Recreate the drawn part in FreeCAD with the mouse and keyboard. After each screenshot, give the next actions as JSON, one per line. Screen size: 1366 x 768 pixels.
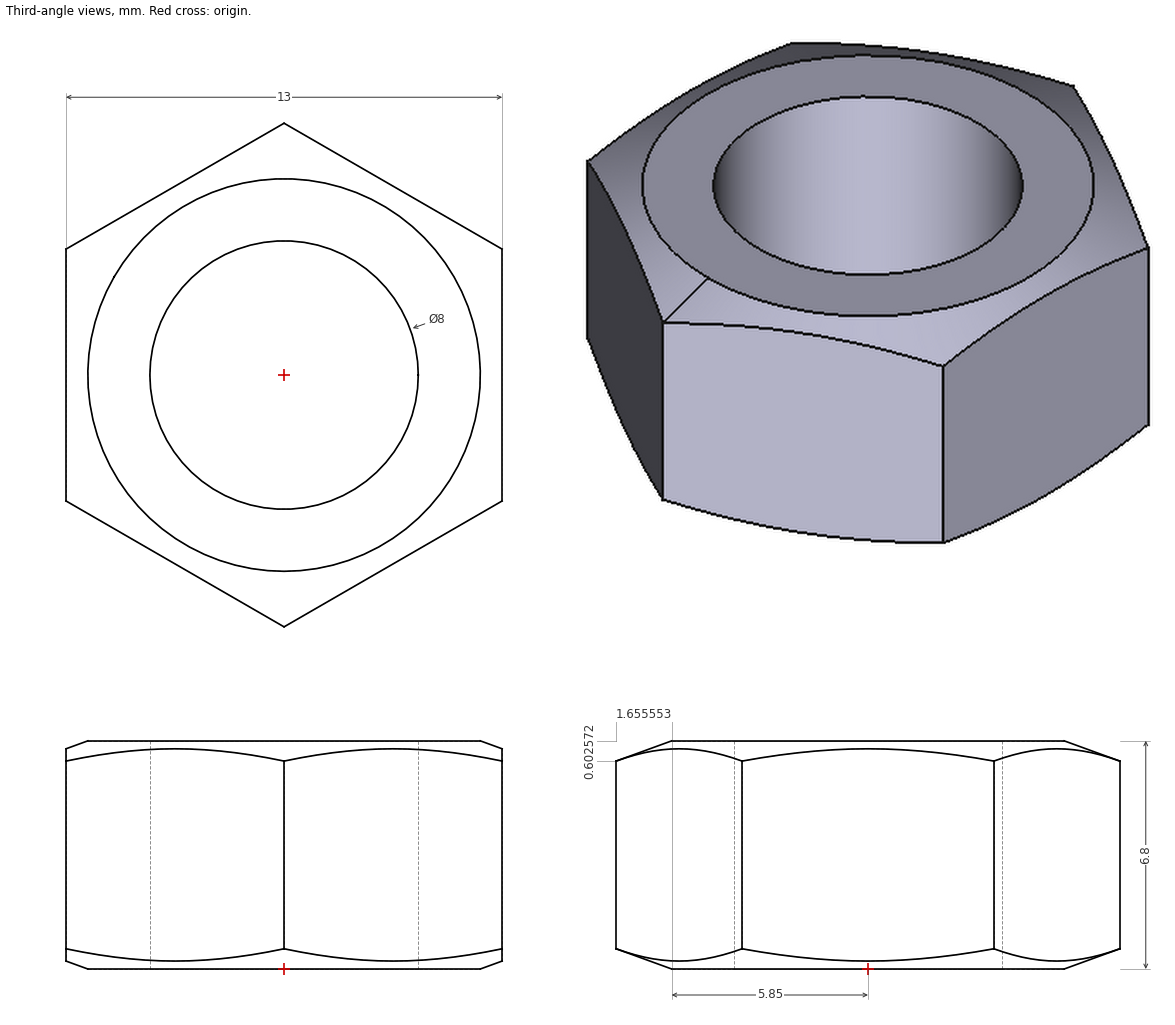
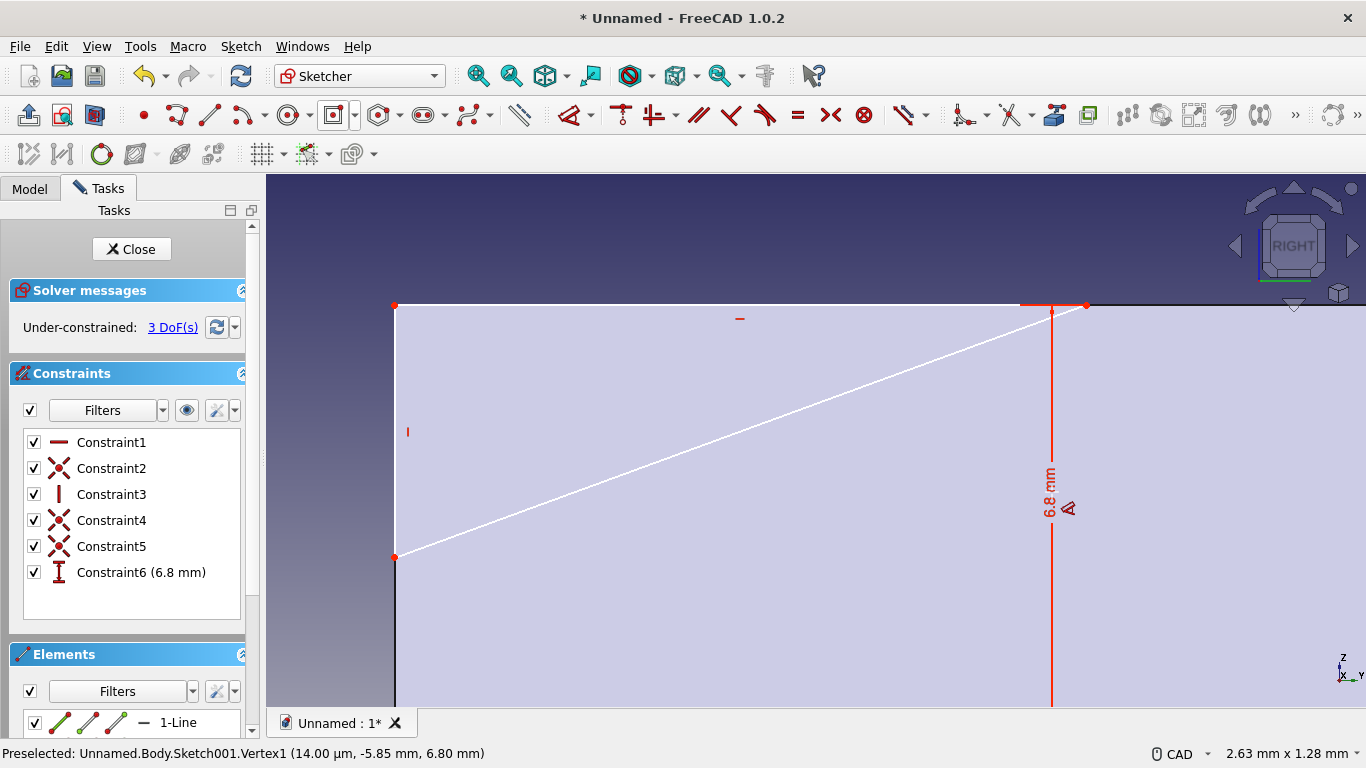
{"action": "left_click", "coordinate": [1086, 305]}
{"action": "left_click", "coordinate": [1143, 271]}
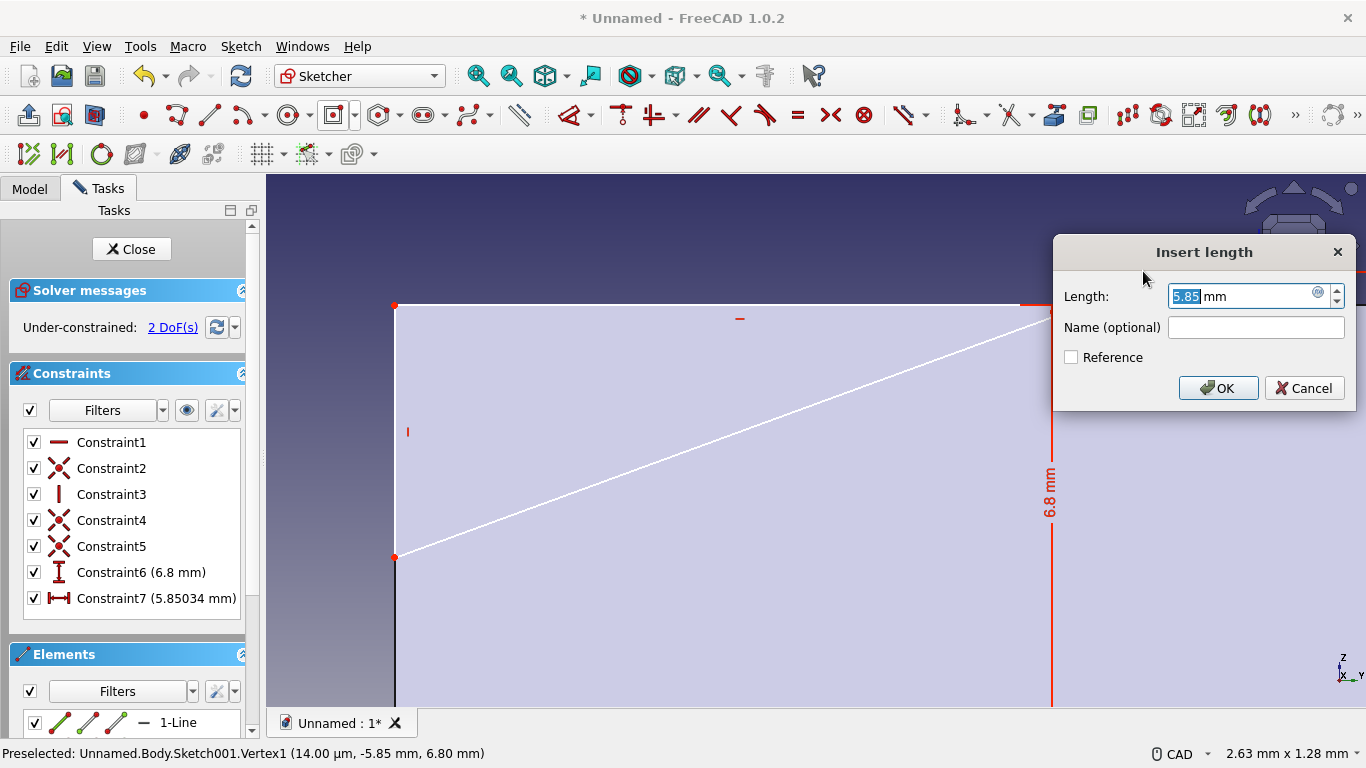
{"action": "type", "text": "5.85"}
{"action": "key", "text": "Return"}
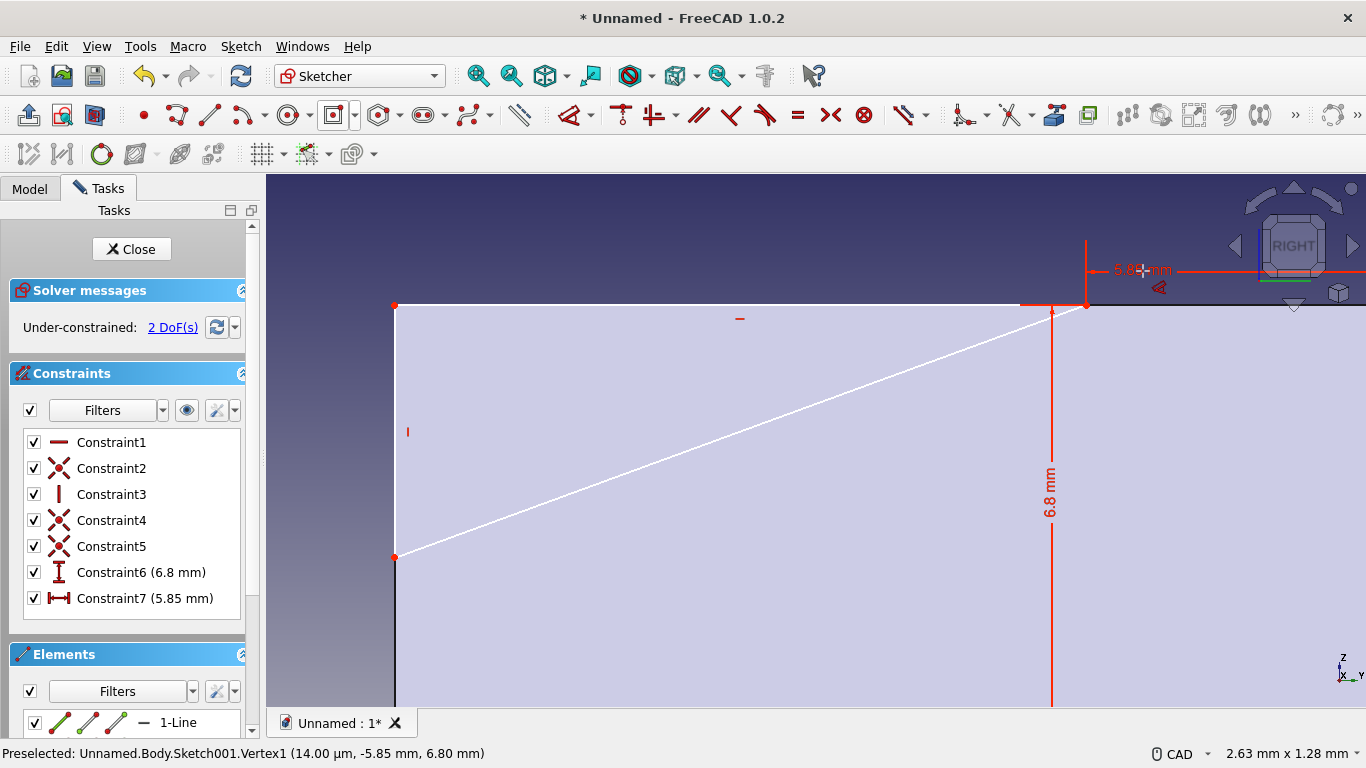
{"action": "left_click", "coordinate": [879, 305]}
{"action": "left_click", "coordinate": [741, 271]}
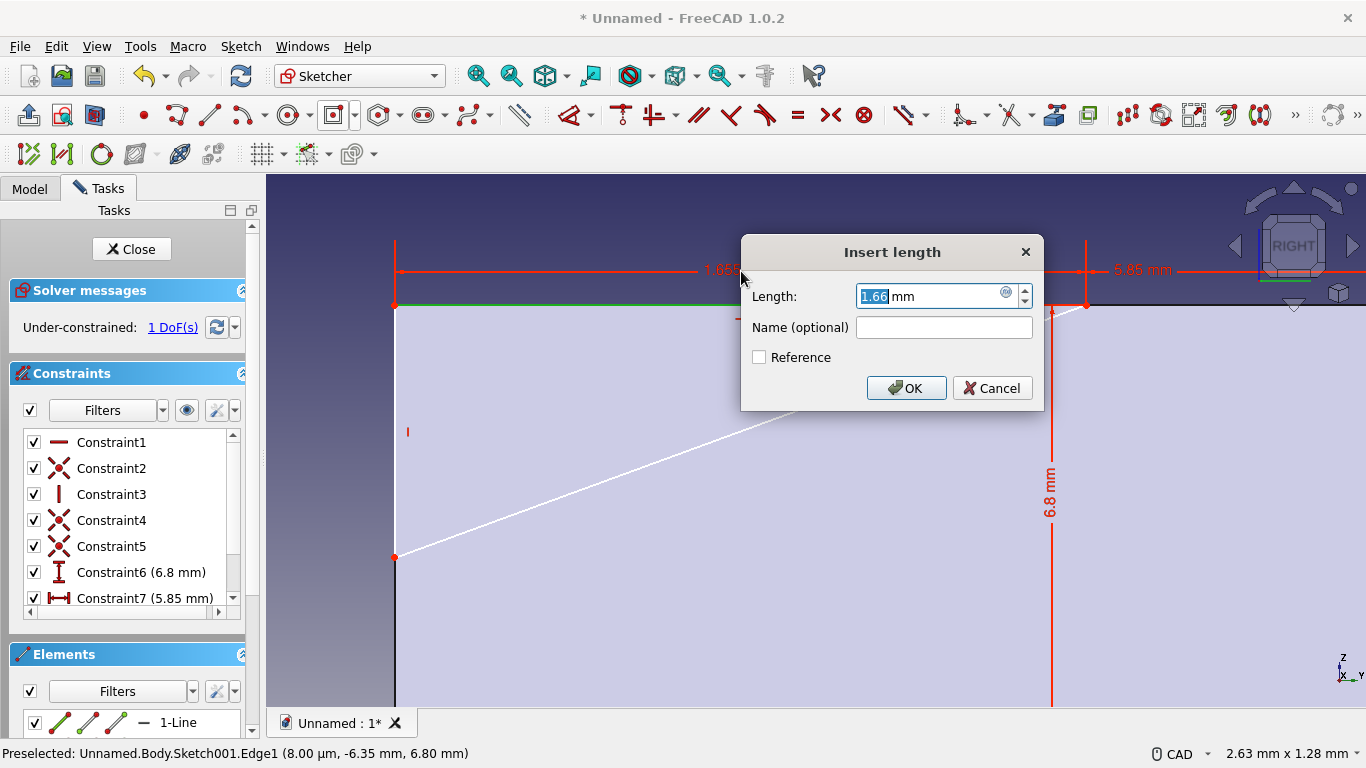
{"action": "type", "text": "1.655553"}
{"action": "key", "text": "Return"}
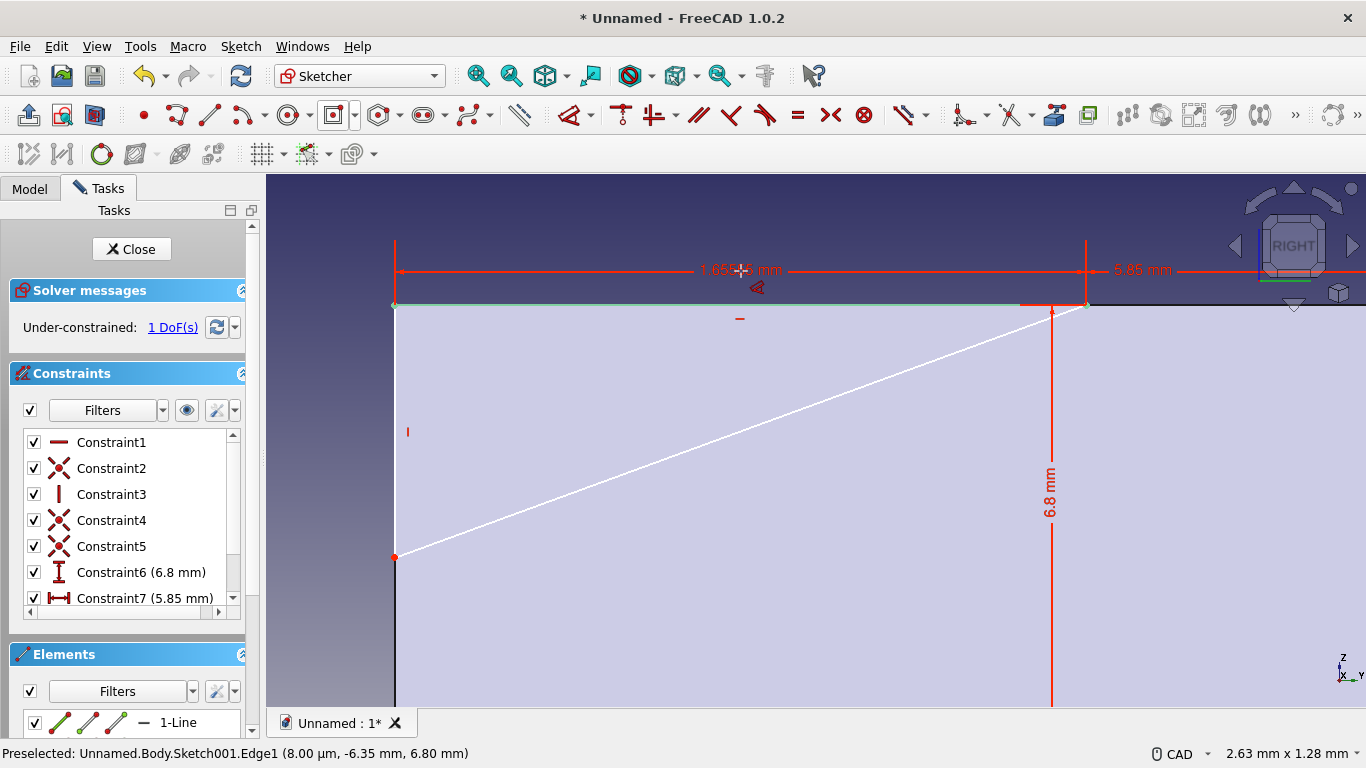
{"action": "left_click", "coordinate": [395, 381]}
{"action": "left_click", "coordinate": [361, 432]}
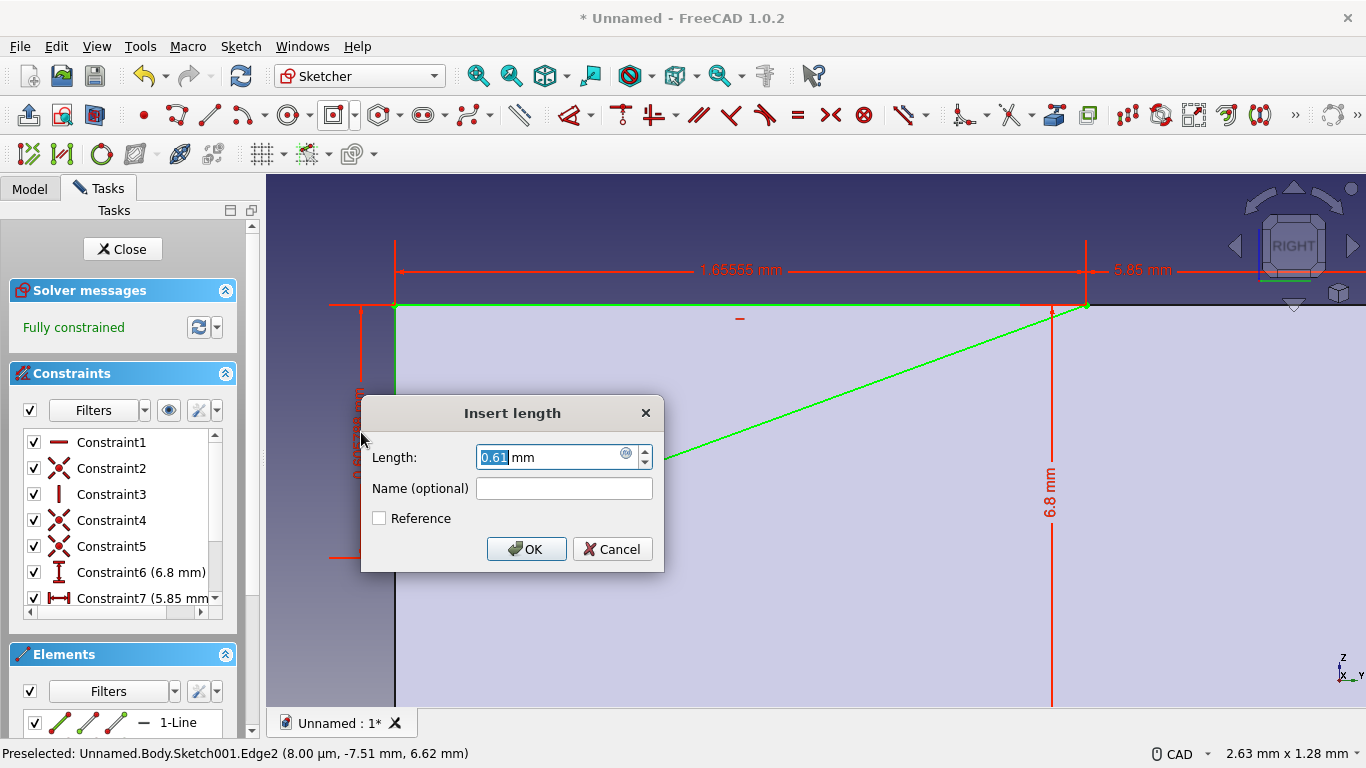
{"action": "type", "text": "0.602572"}
{"action": "key", "text": "Return"}
{"action": "key", "text": "Escape"}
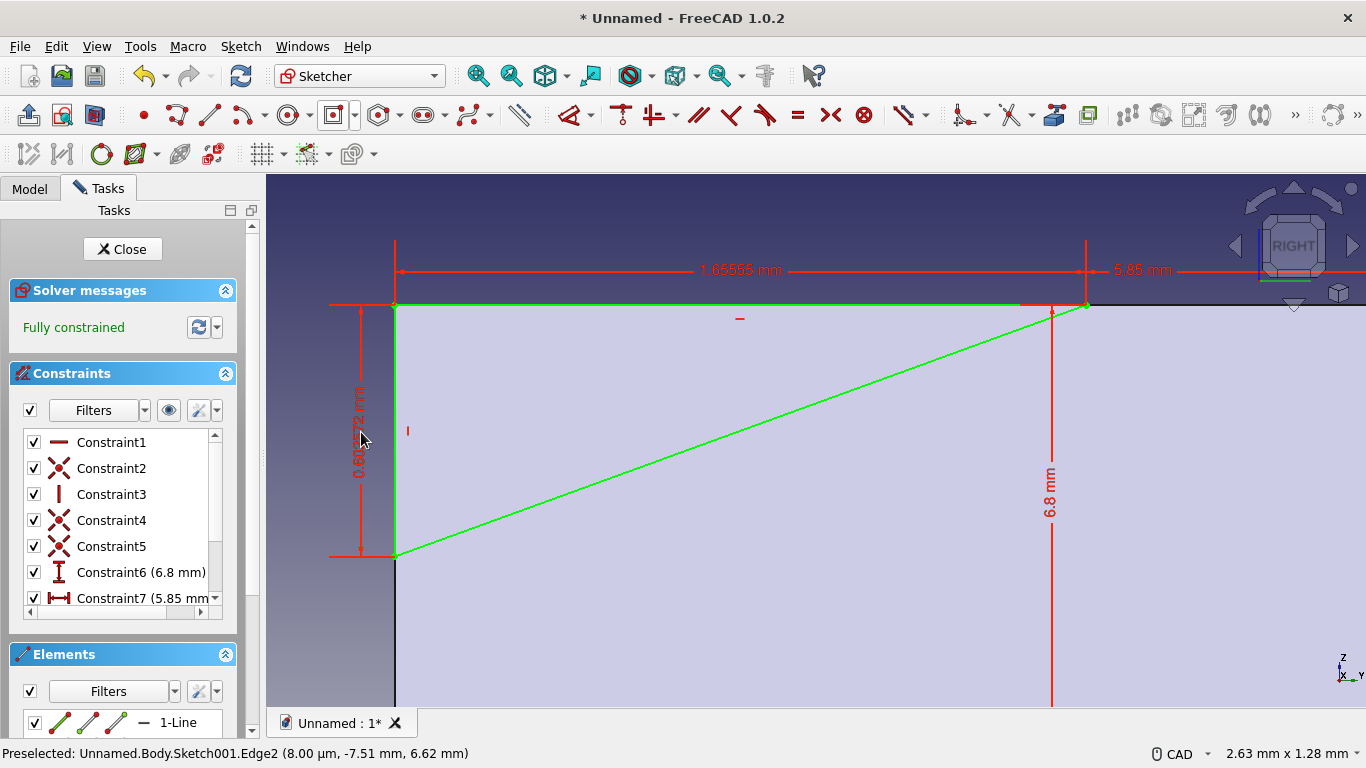
{"action": "left_click", "coordinate": [123, 249]}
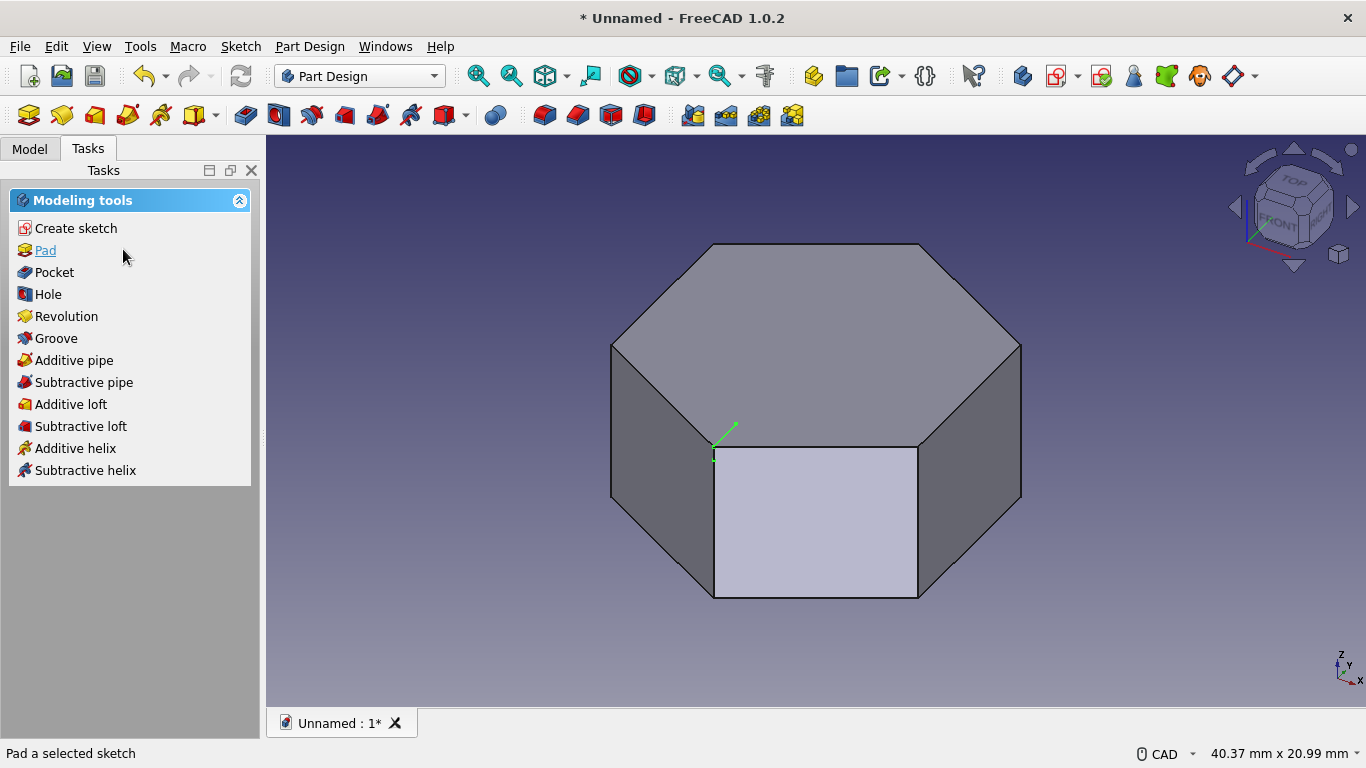
{"action": "left_click", "coordinate": [312, 116]}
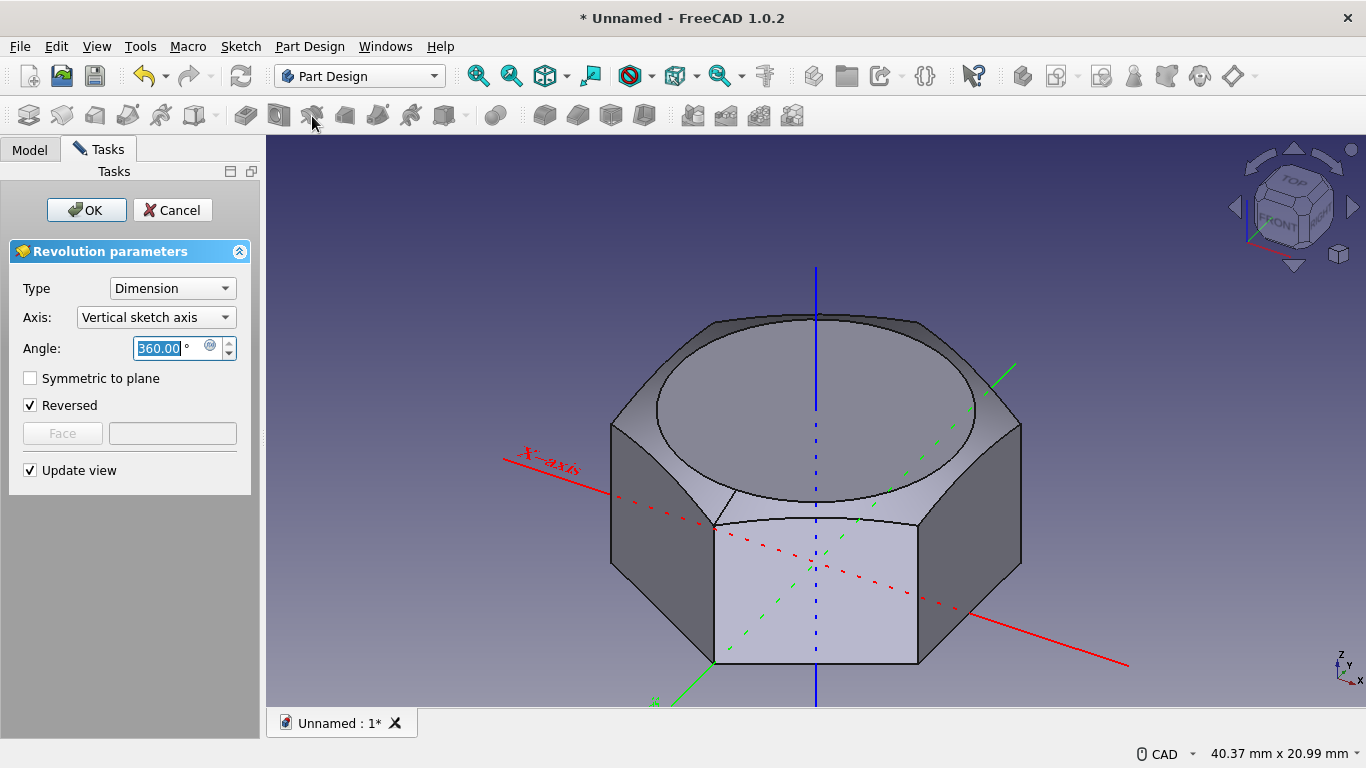
{"action": "left_click", "coordinate": [87, 210]}